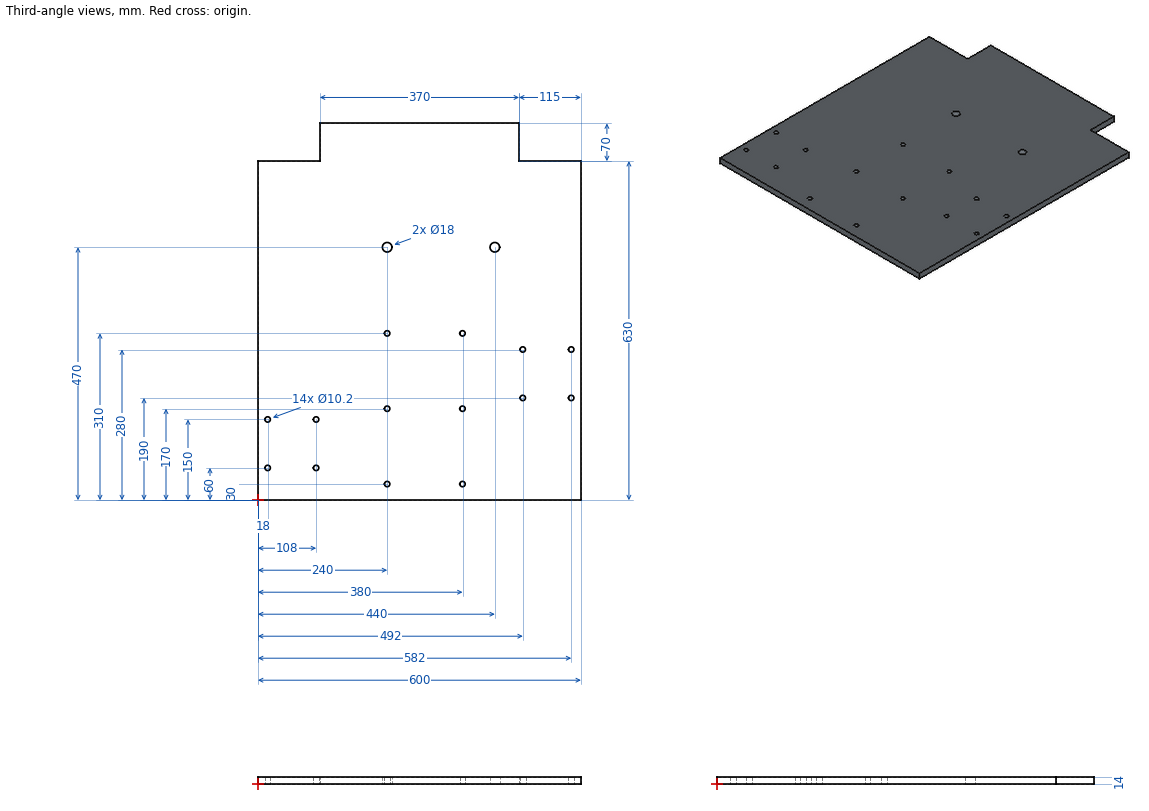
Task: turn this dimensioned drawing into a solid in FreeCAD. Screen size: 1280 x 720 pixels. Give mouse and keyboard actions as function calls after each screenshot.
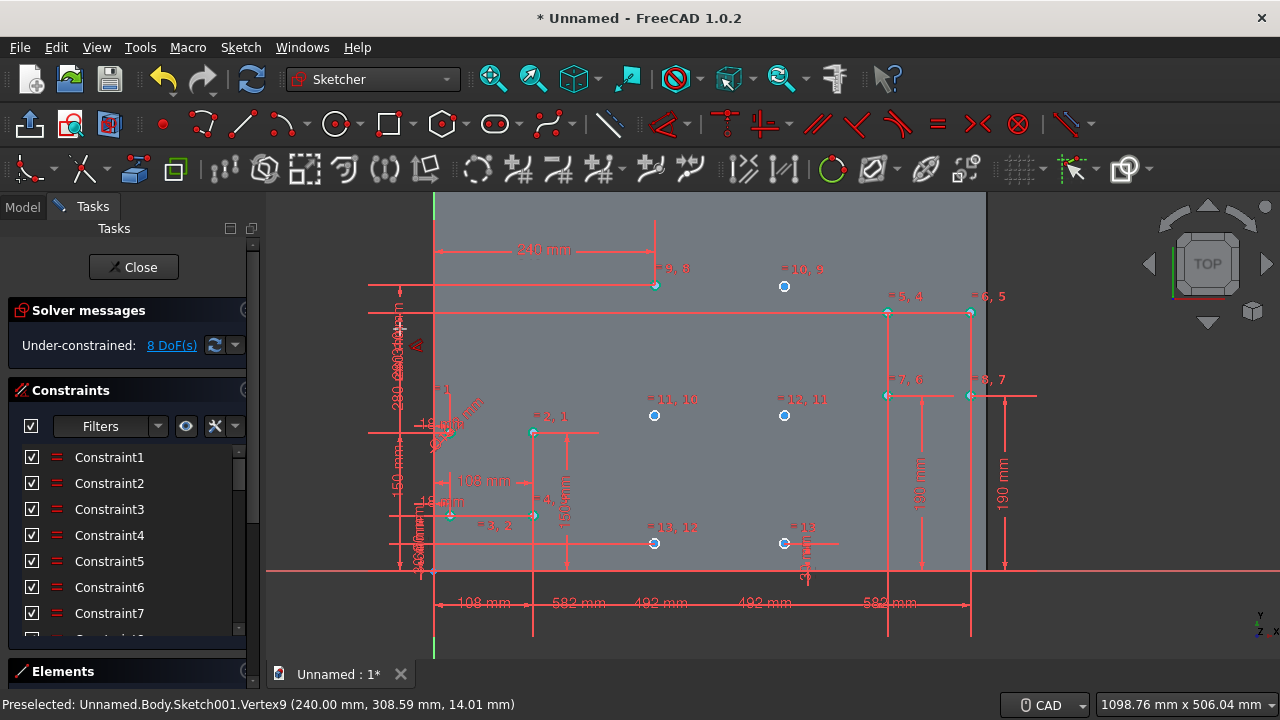
click(785, 286)
click(690, 252)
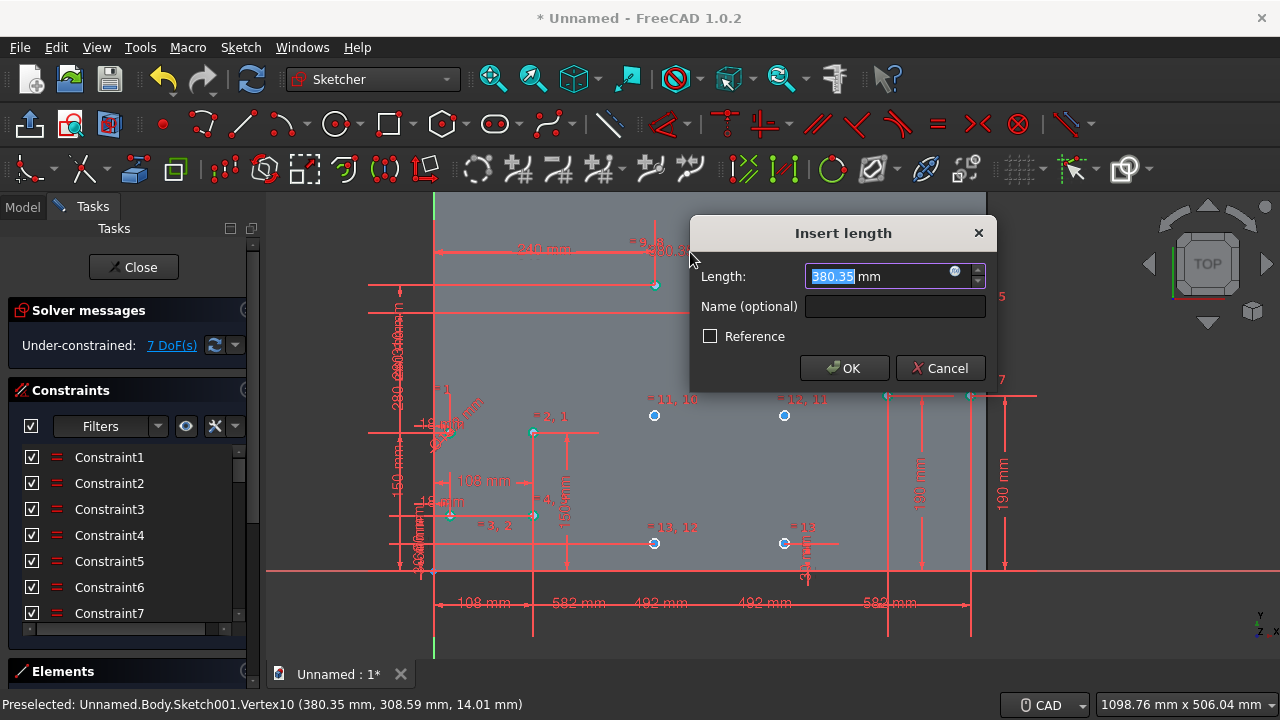
text(380)
key(Return)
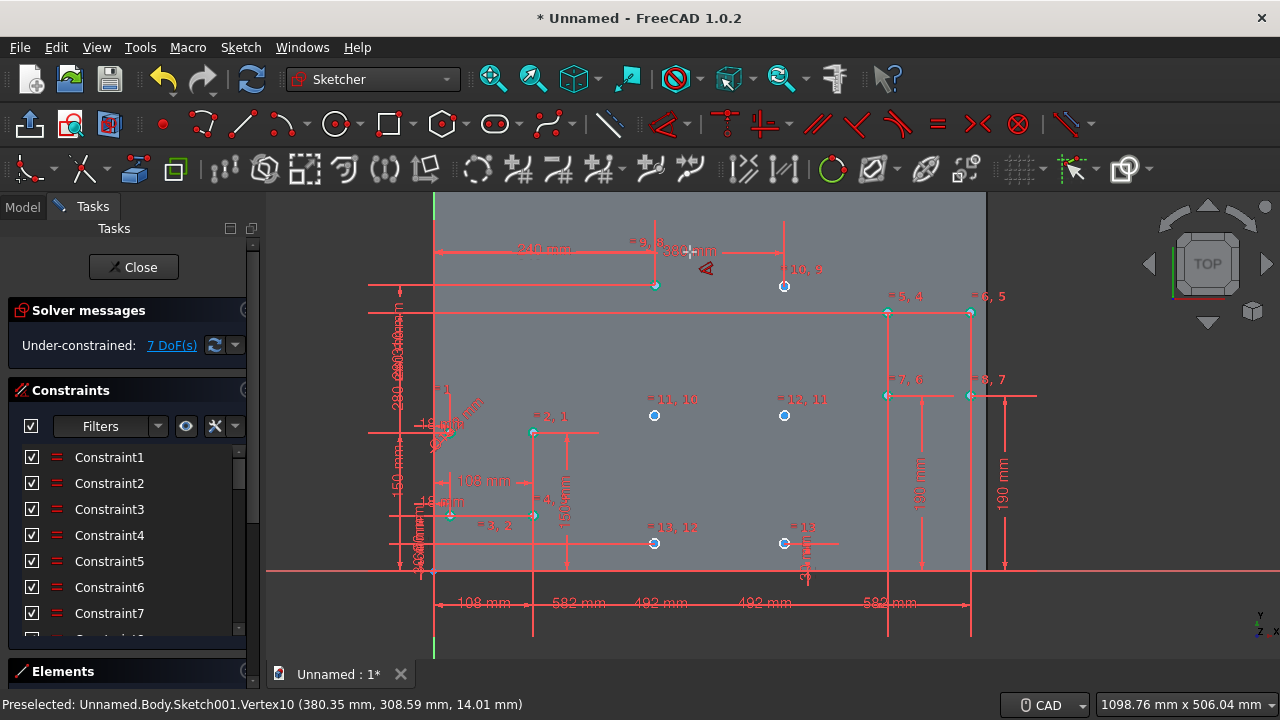
click(784, 286)
click(818, 429)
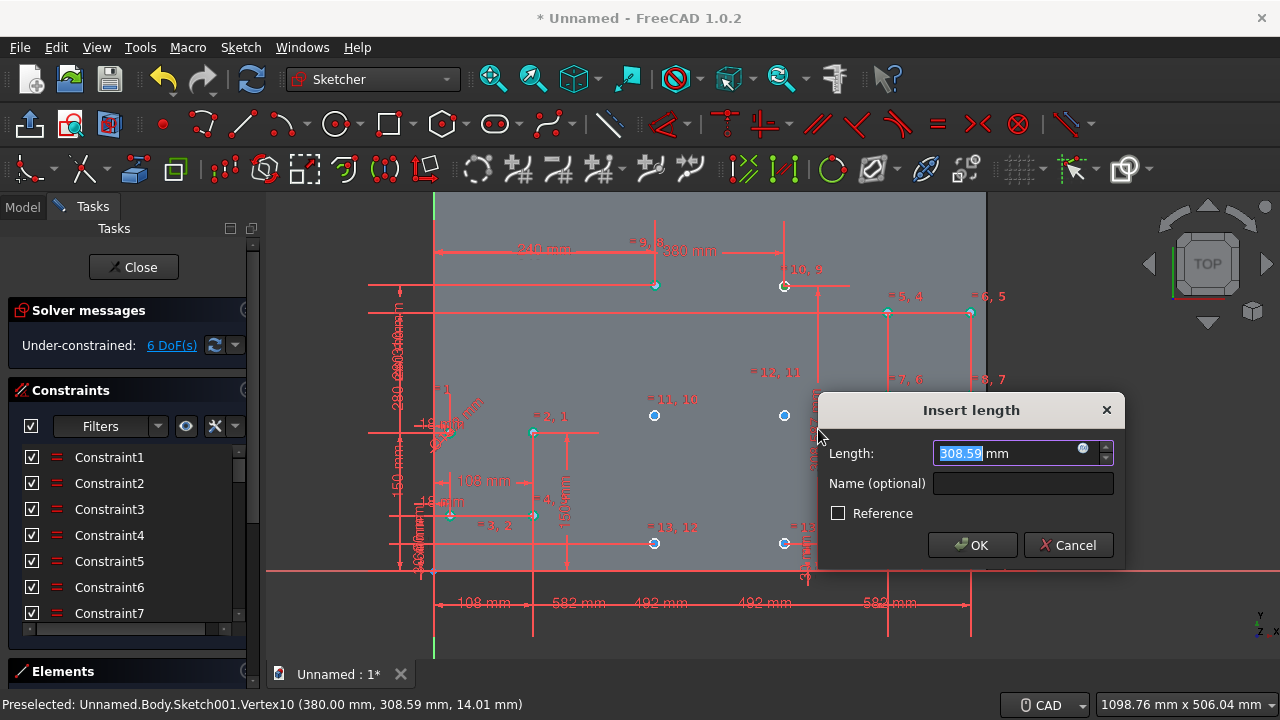
text(310)
key(Return)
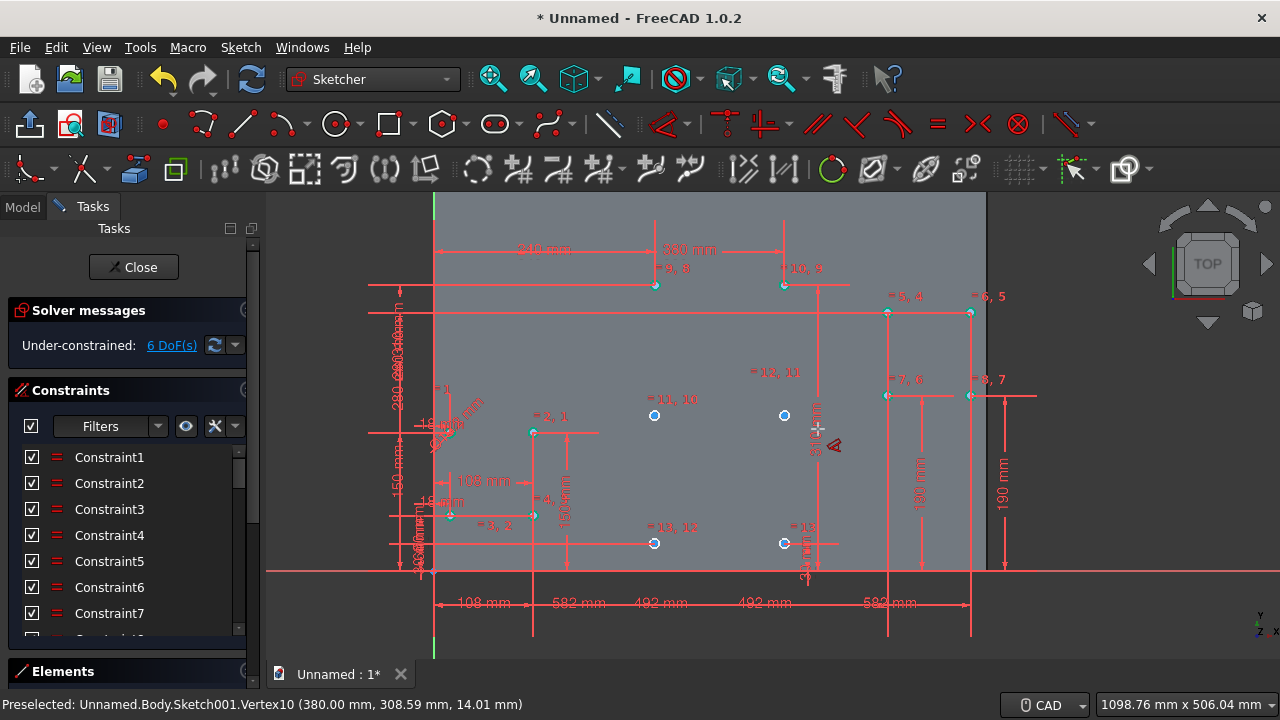
click(655, 416)
click(544, 382)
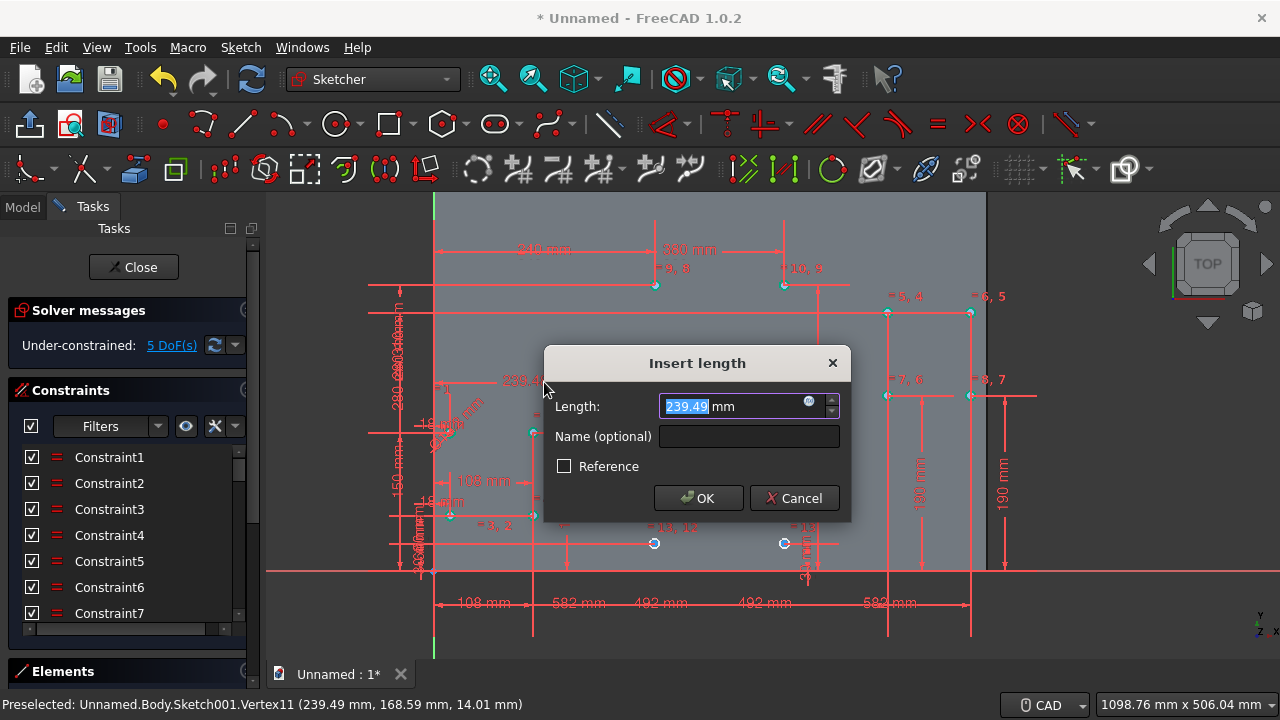
text(240)
key(Return)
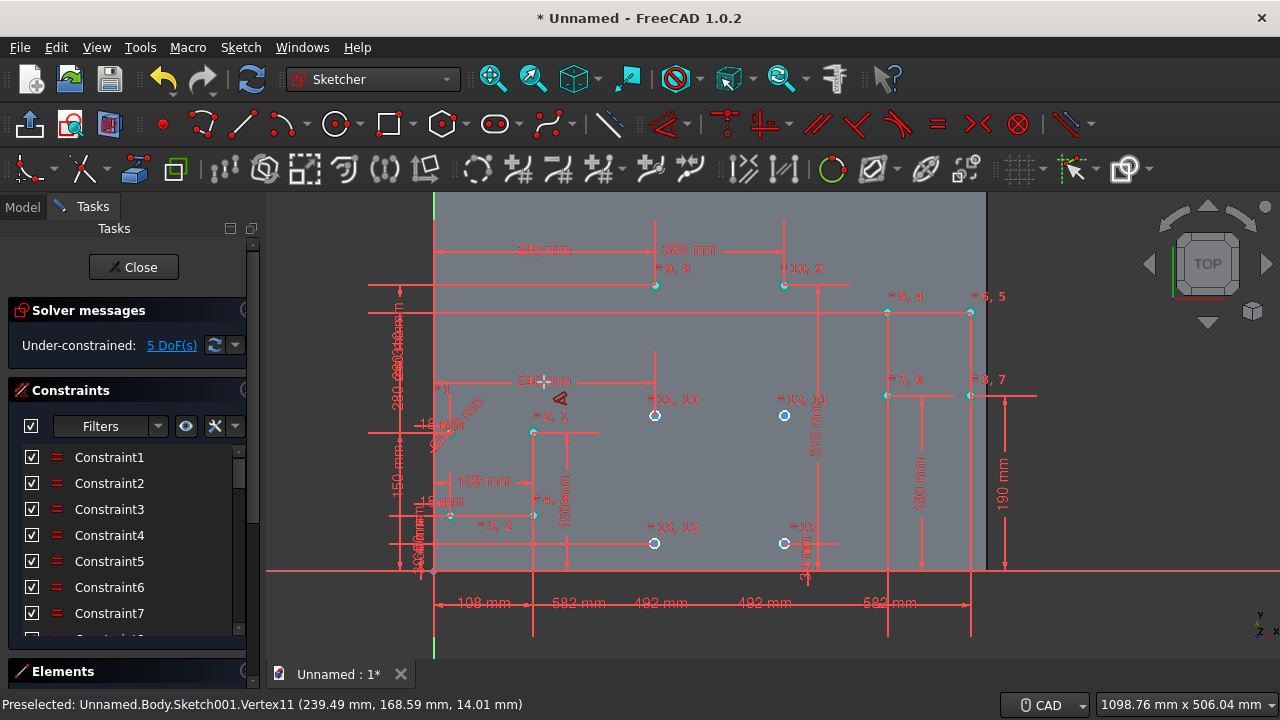
click(655, 416)
click(689, 493)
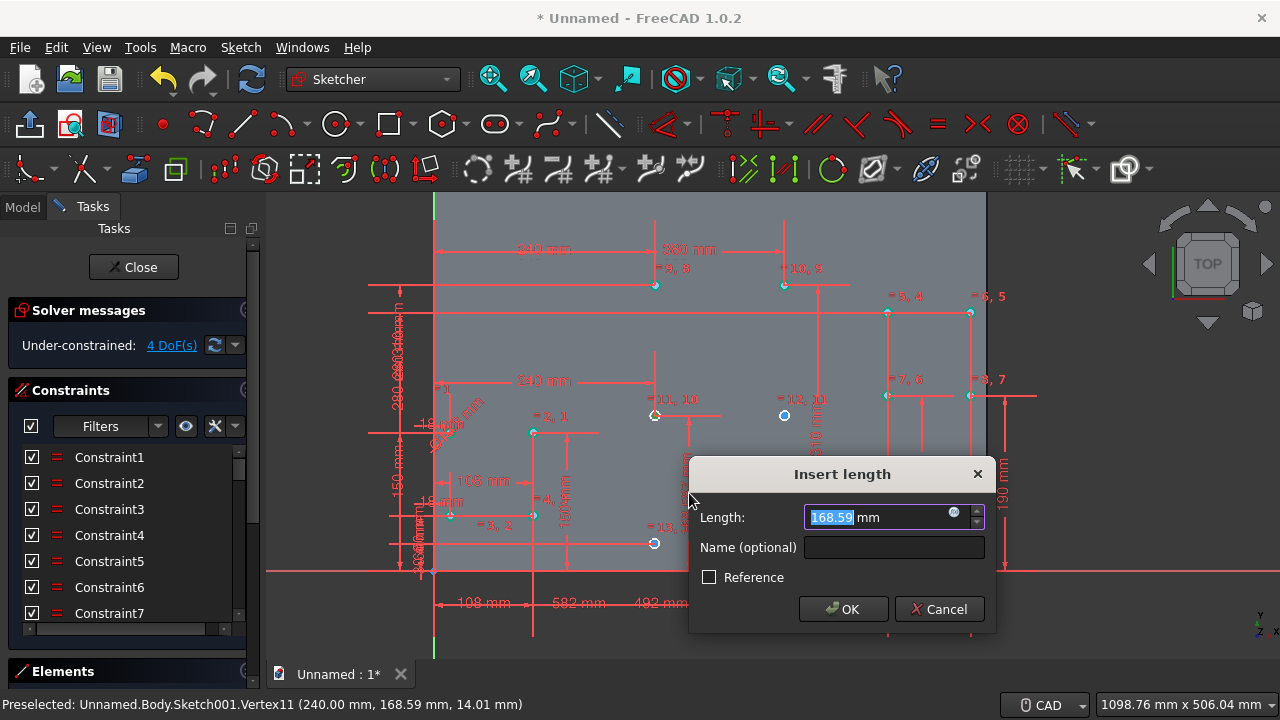
text(170)
key(Return)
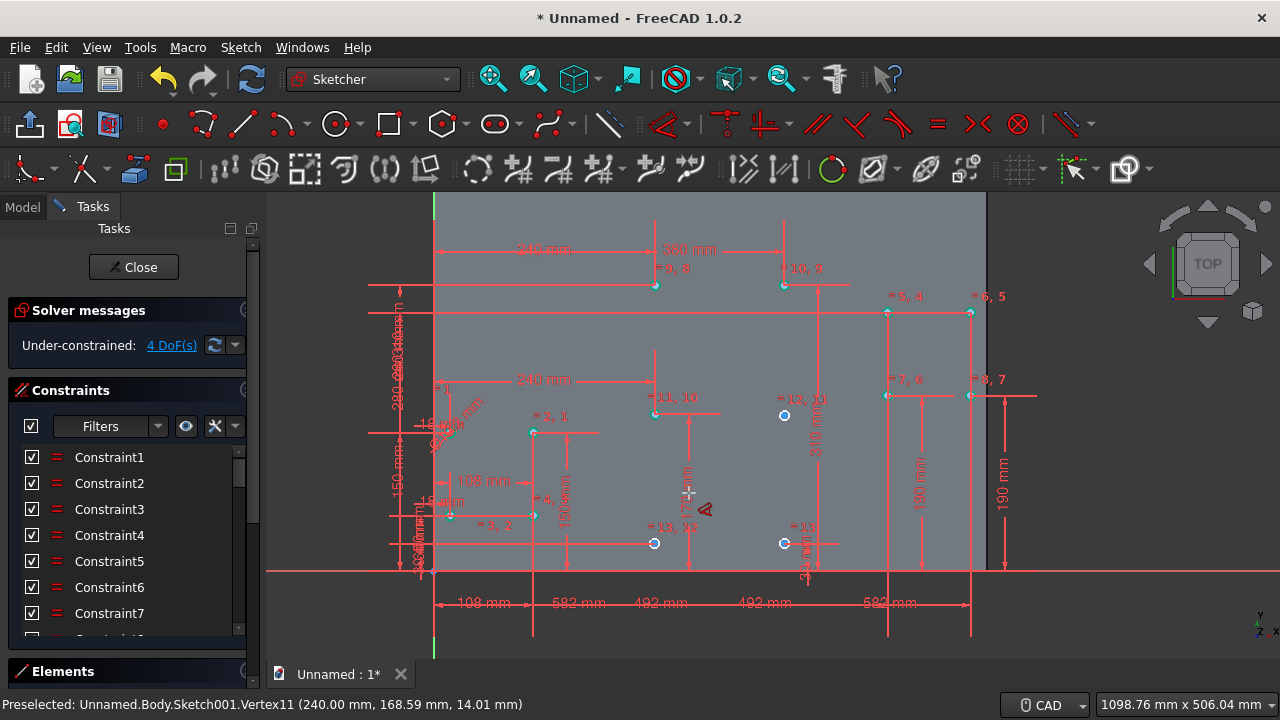
click(785, 416)
click(690, 382)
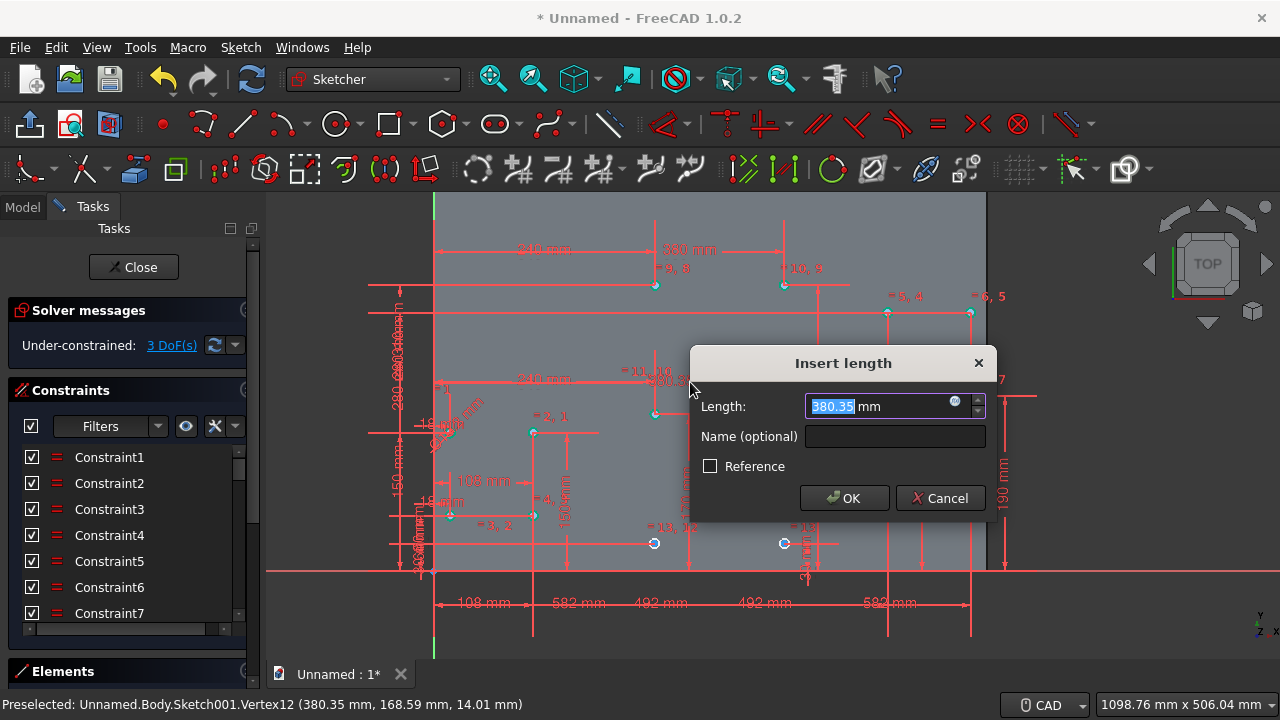
text(380)
key(Return)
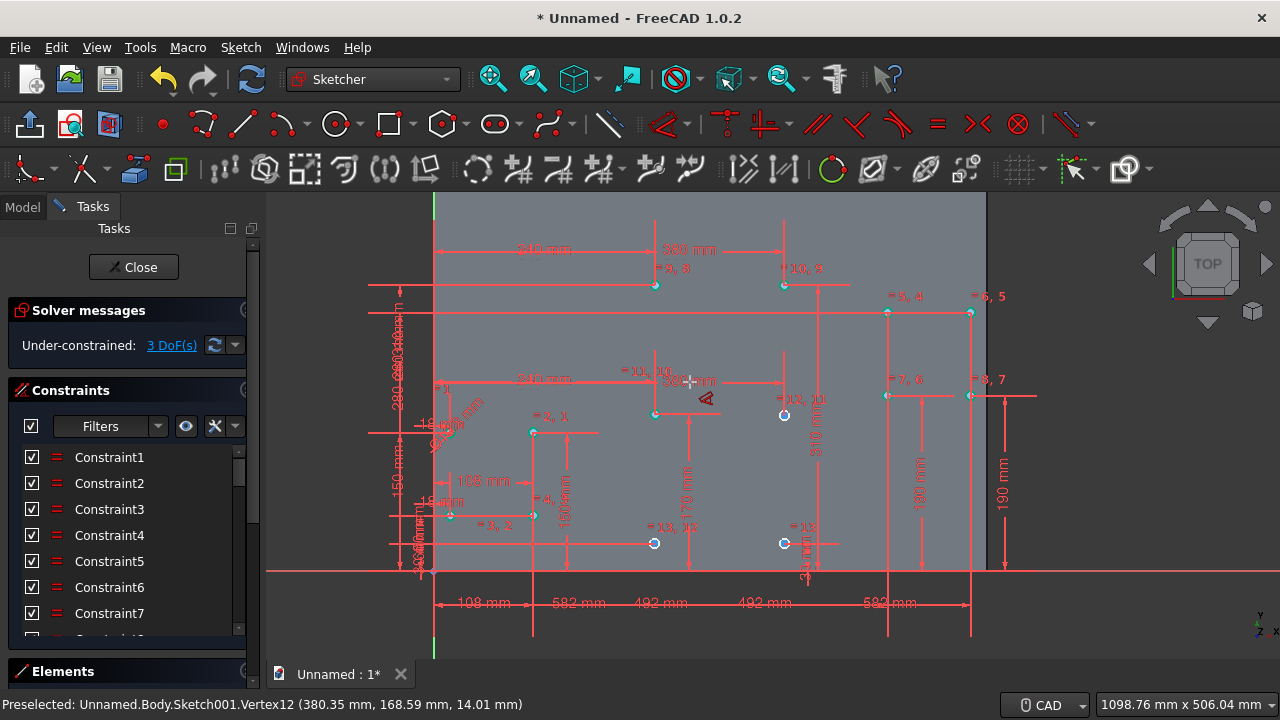
click(784, 416)
click(818, 493)